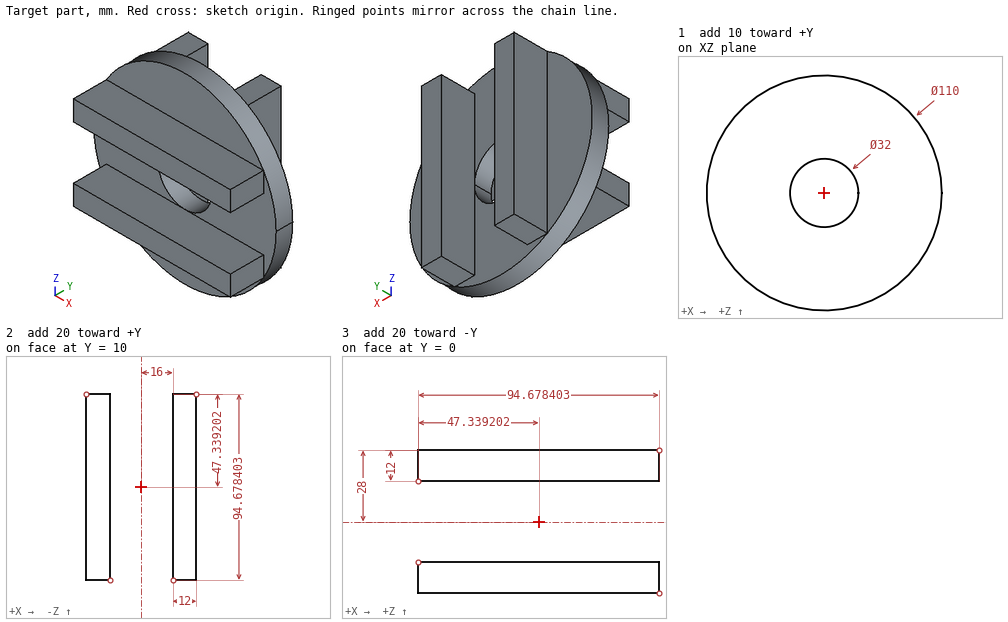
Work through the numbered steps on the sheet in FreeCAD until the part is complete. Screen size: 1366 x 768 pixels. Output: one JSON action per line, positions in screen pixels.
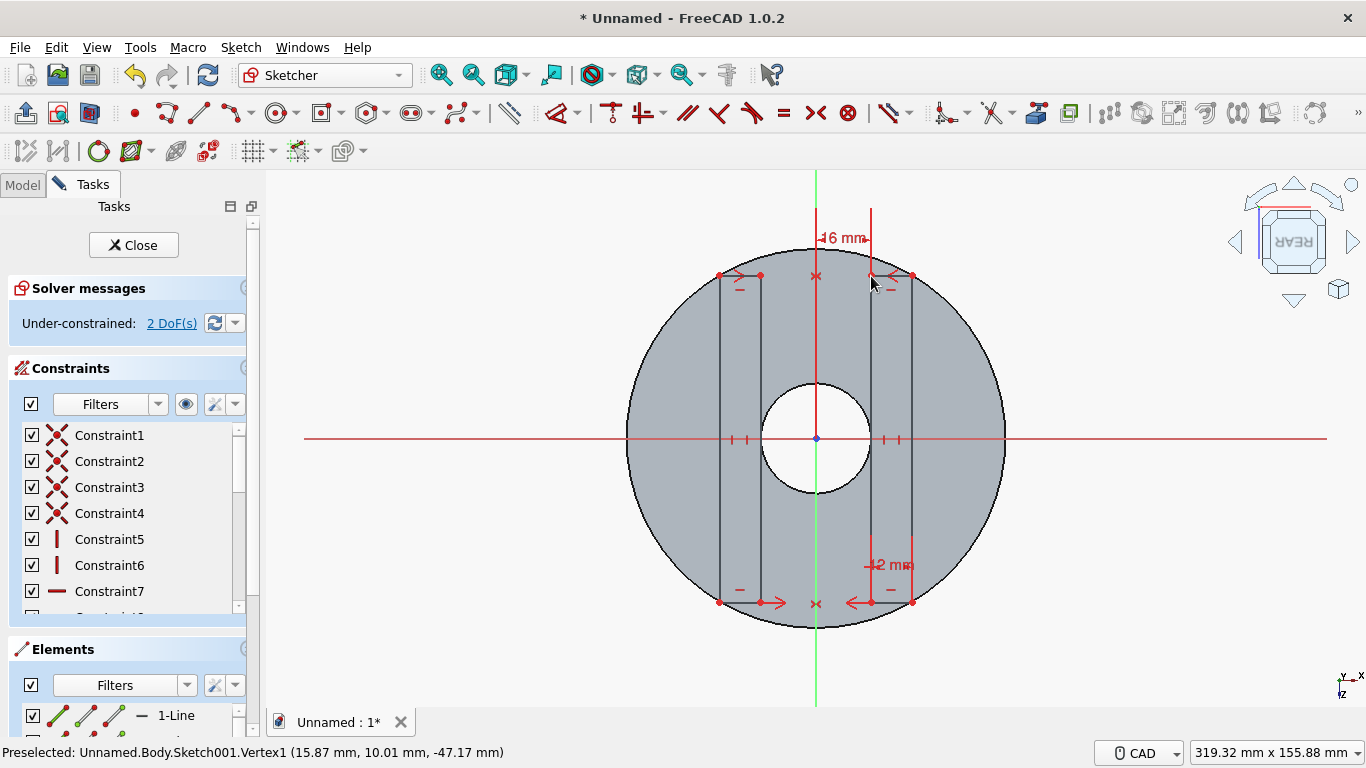
{"action": "left_click", "coordinate": [871, 374]}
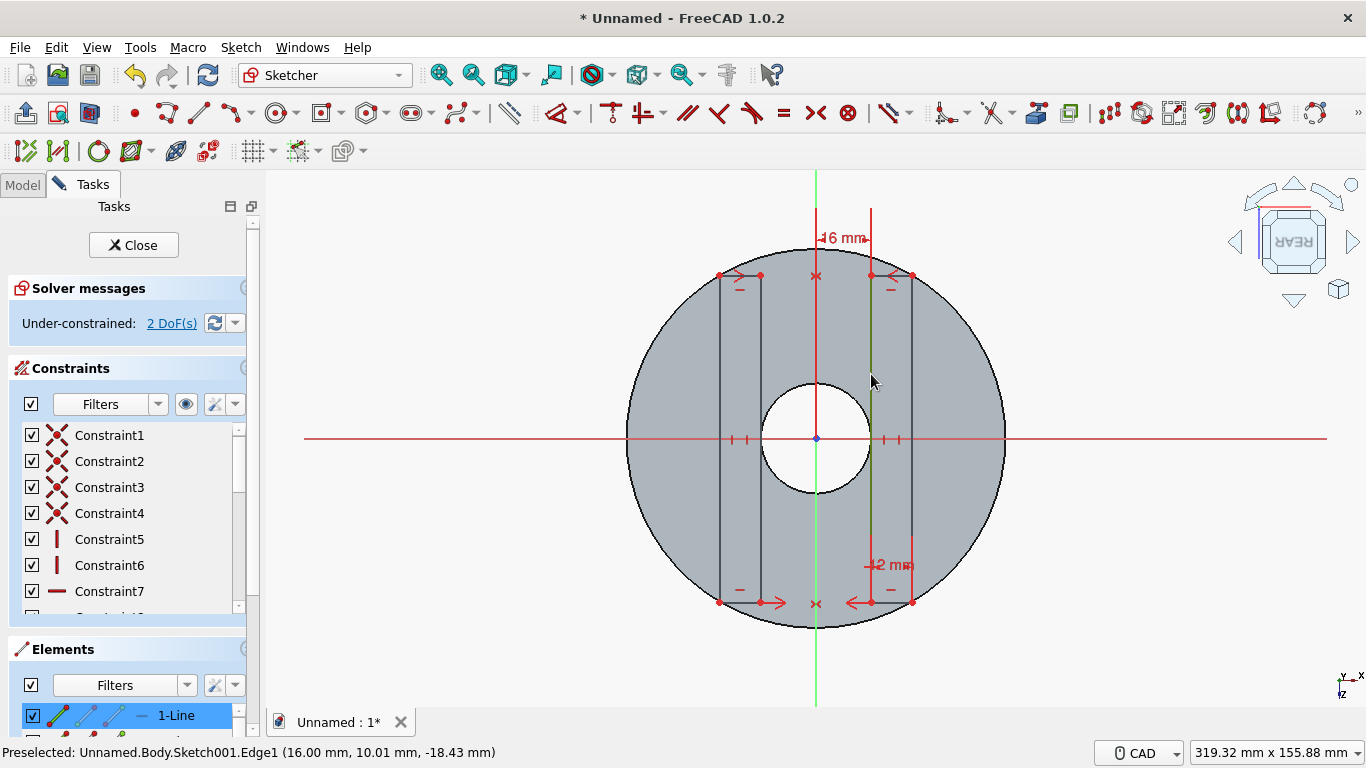
{"action": "key", "text": "i"}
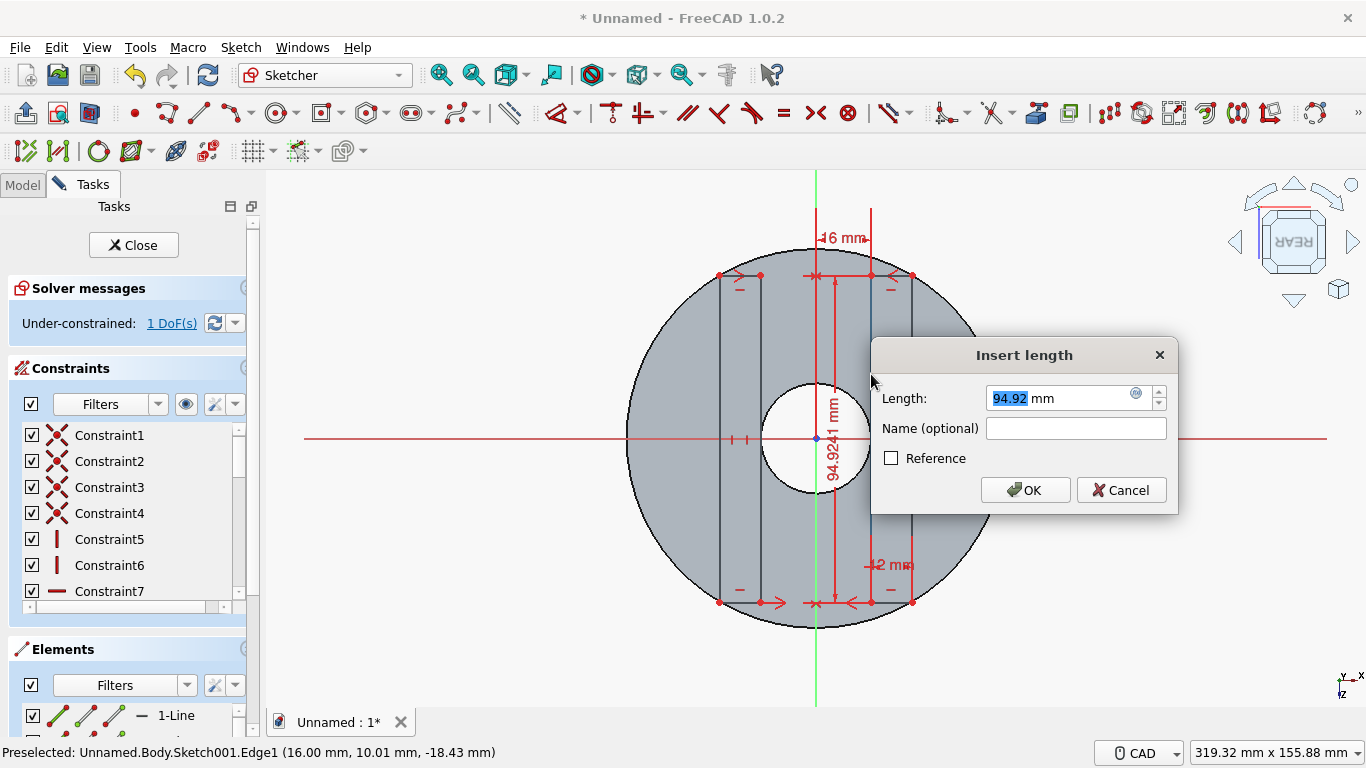
{"action": "type", "text": "94.678403"}
{"action": "key", "text": "Return"}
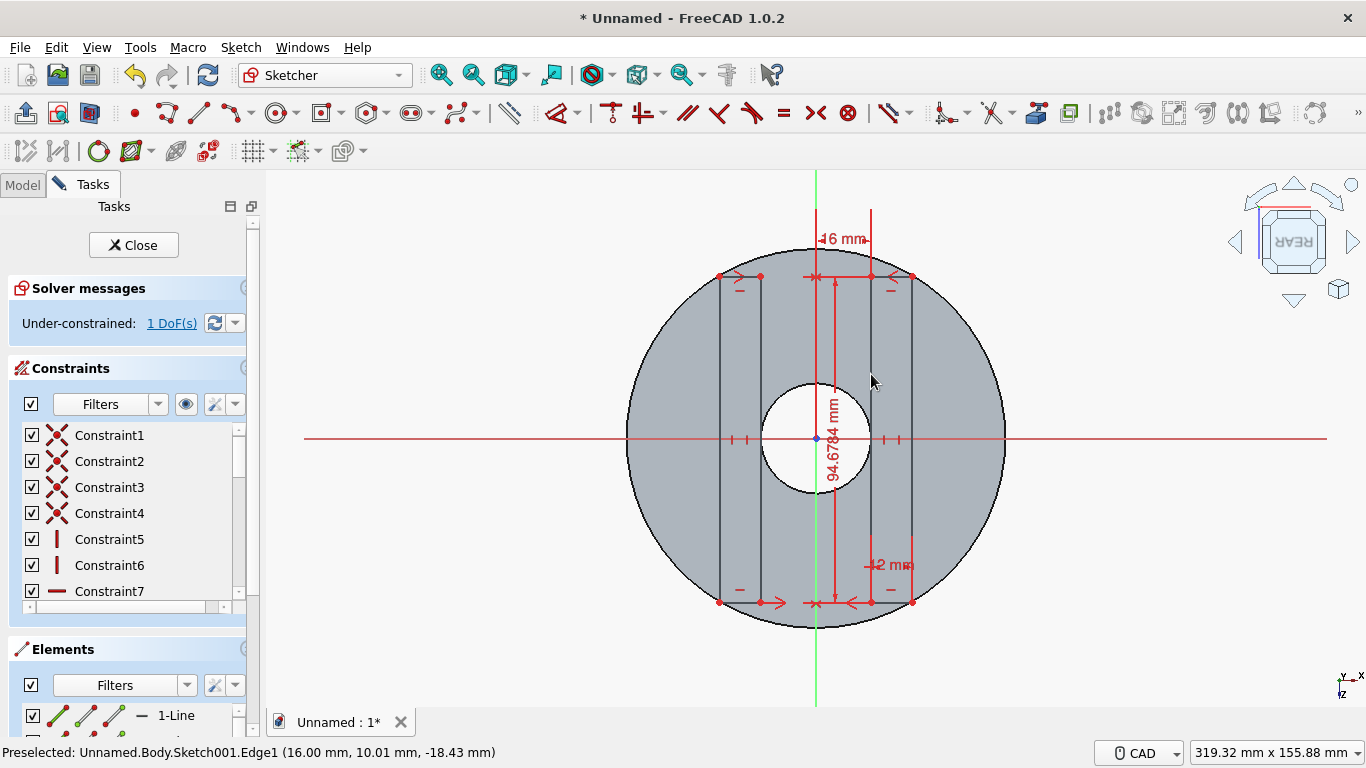
{"action": "left_click", "coordinate": [871, 277]}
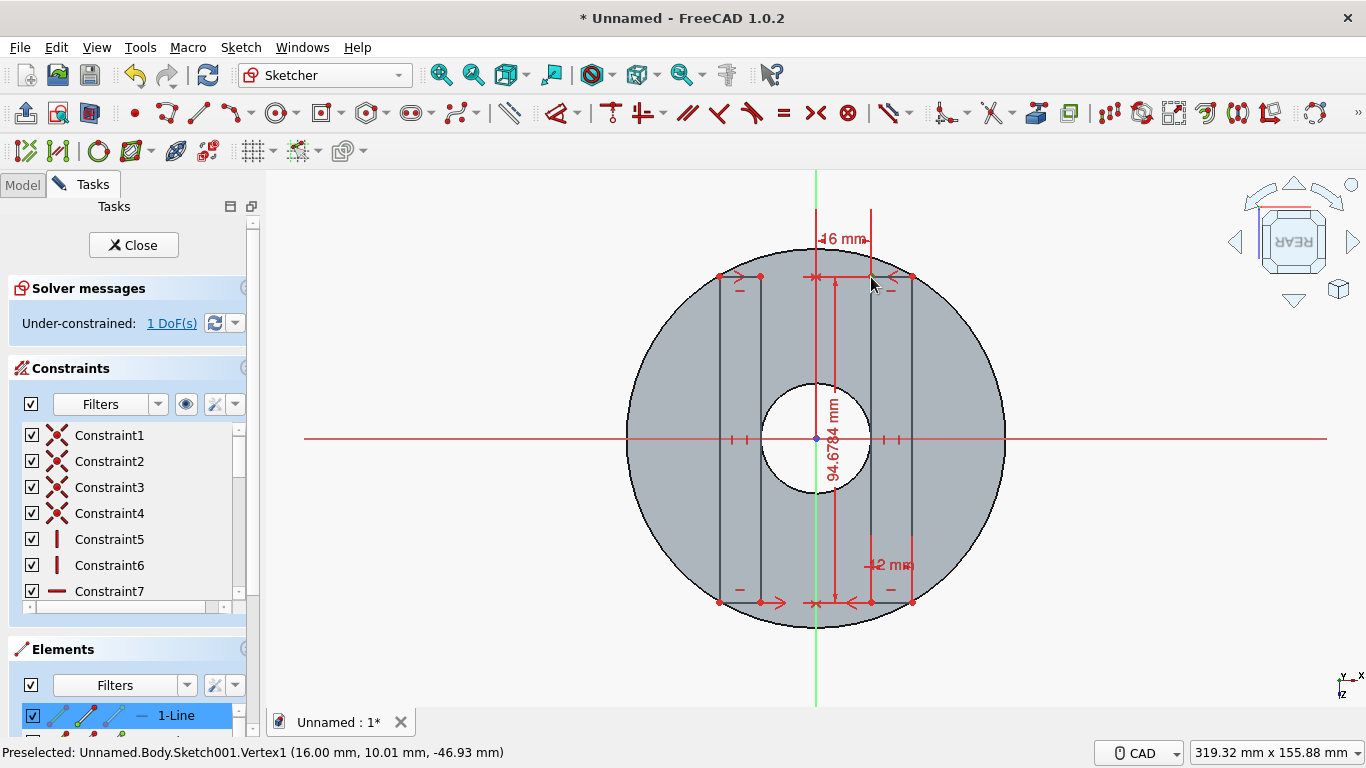
{"action": "key", "text": "i"}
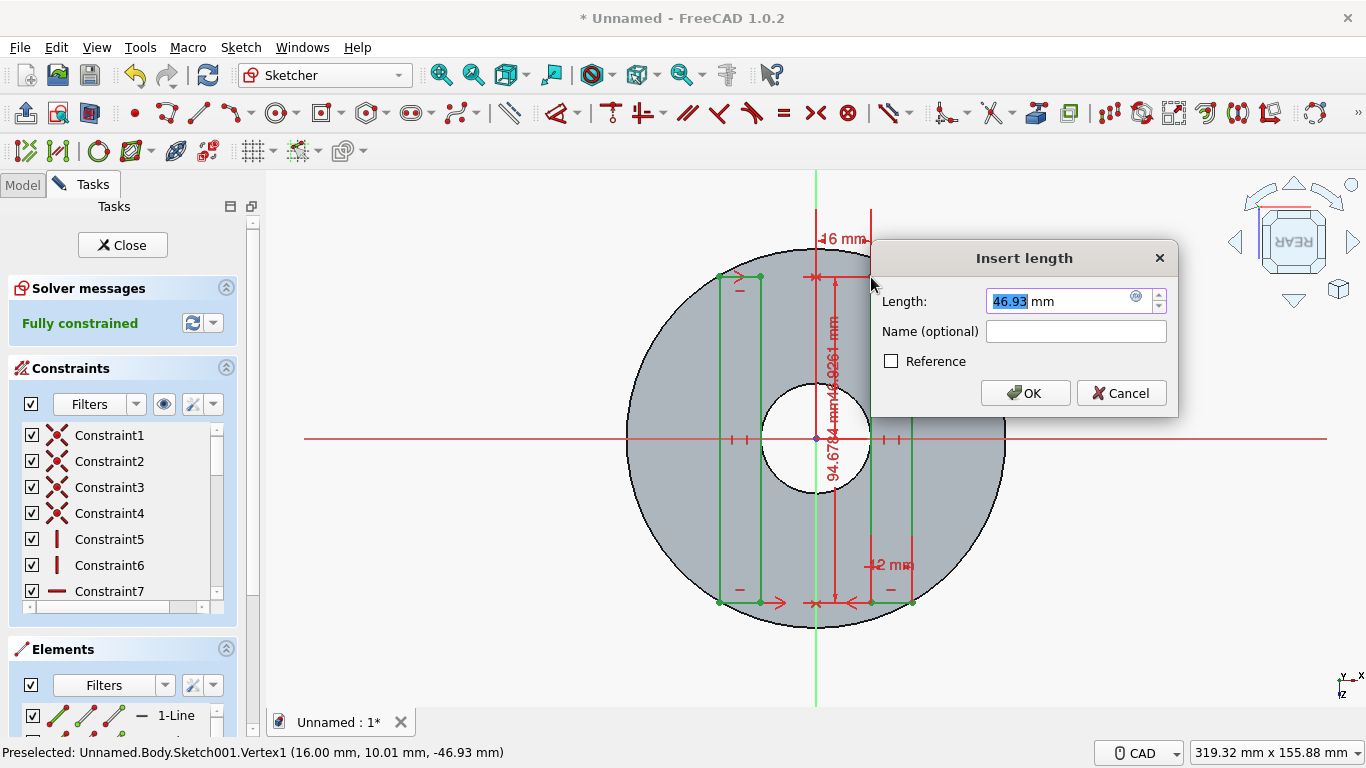
{"action": "type", "text": "47.339202"}
{"action": "key", "text": "Return"}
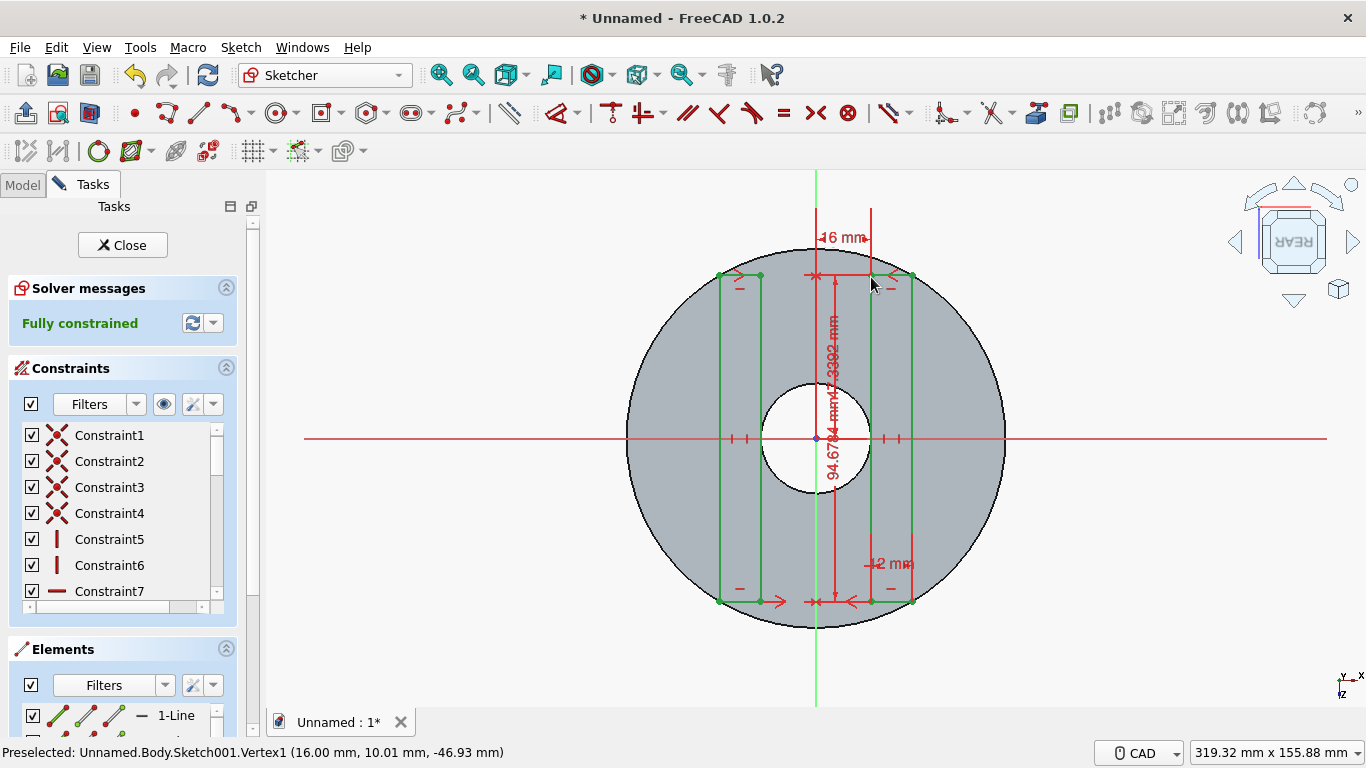
{"action": "left_click", "coordinate": [123, 245]}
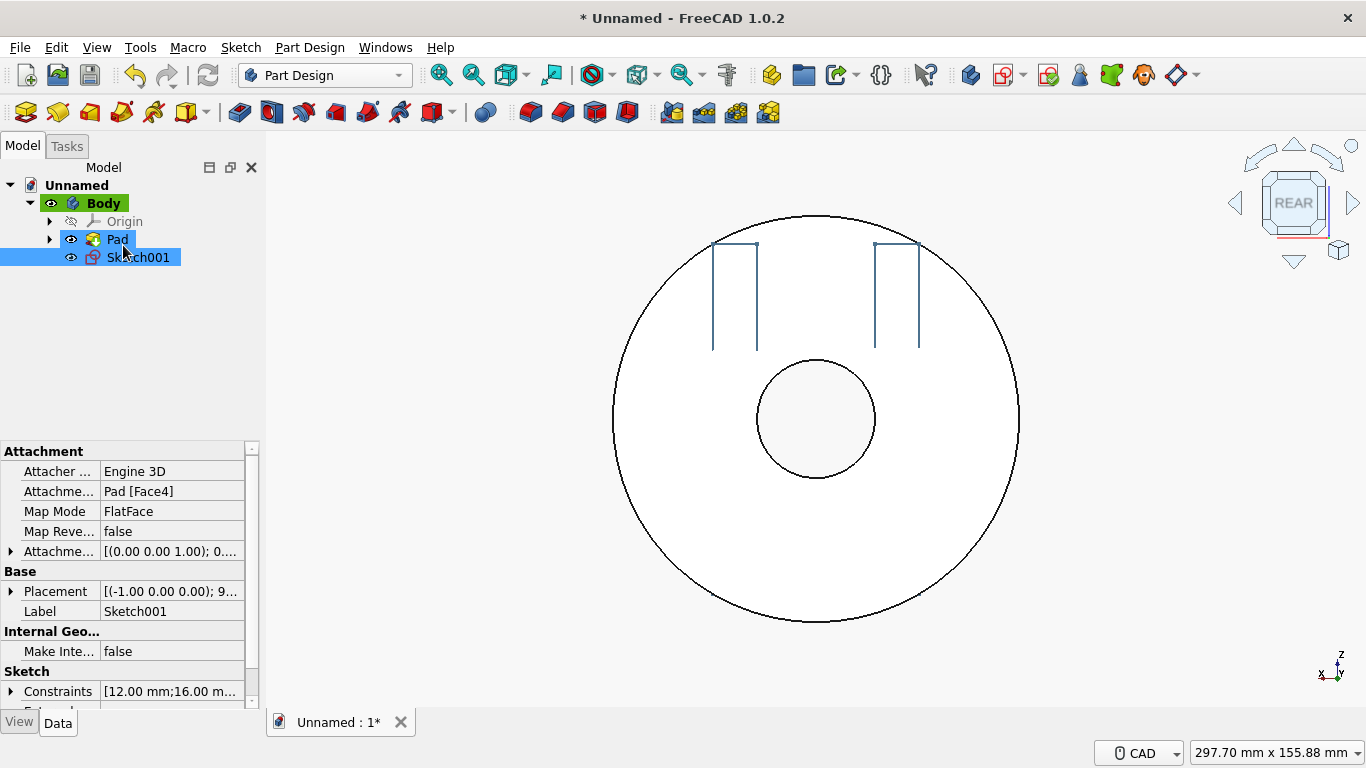
{"action": "left_click", "coordinate": [26, 112]}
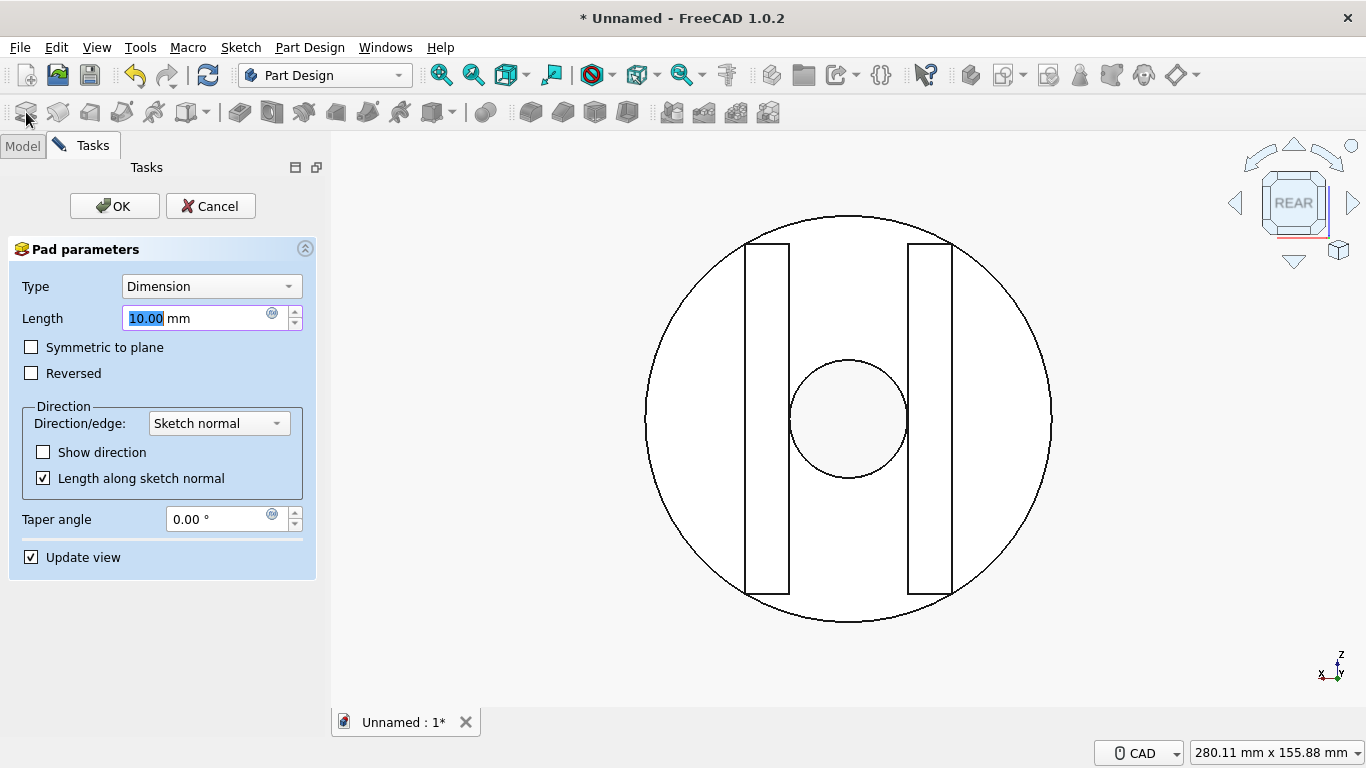
{"action": "type", "text": "20"}
{"action": "key", "text": "Tab"}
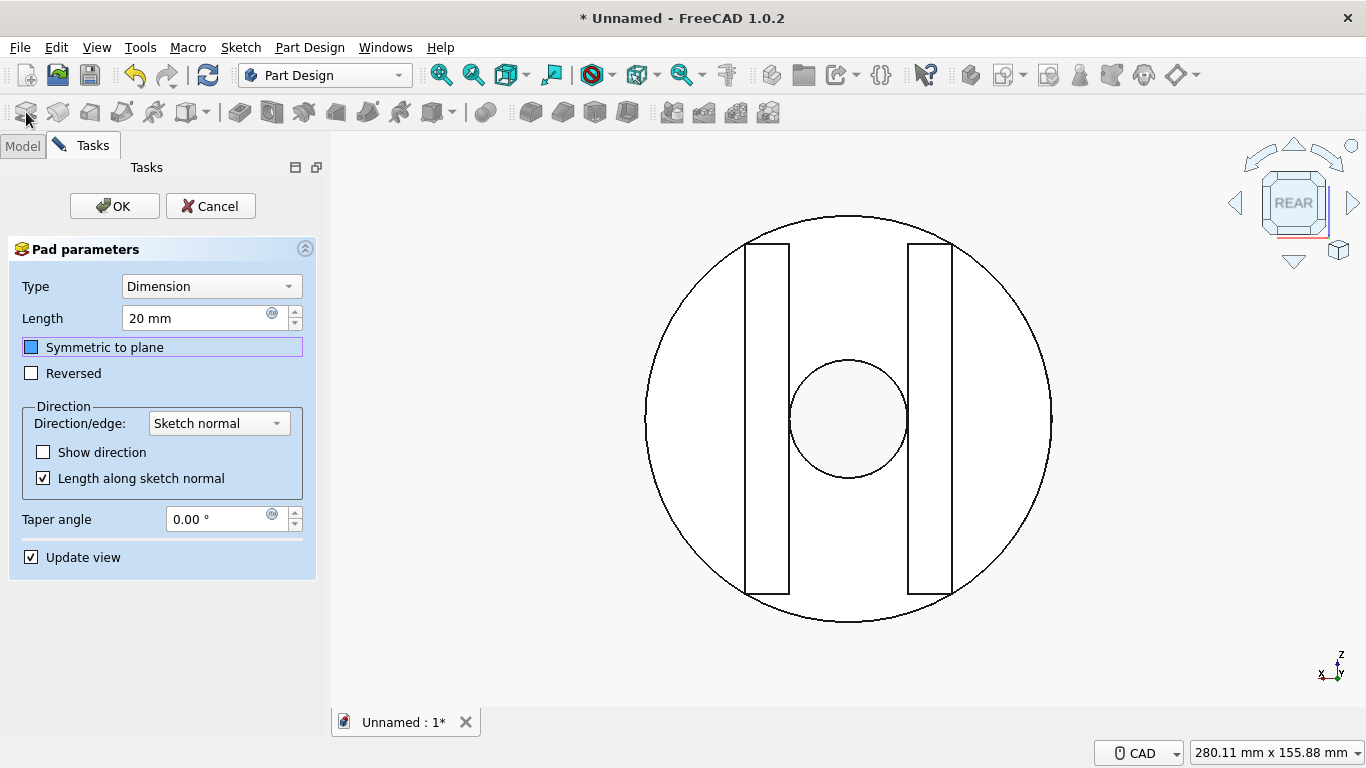
{"action": "left_click", "coordinate": [115, 206]}